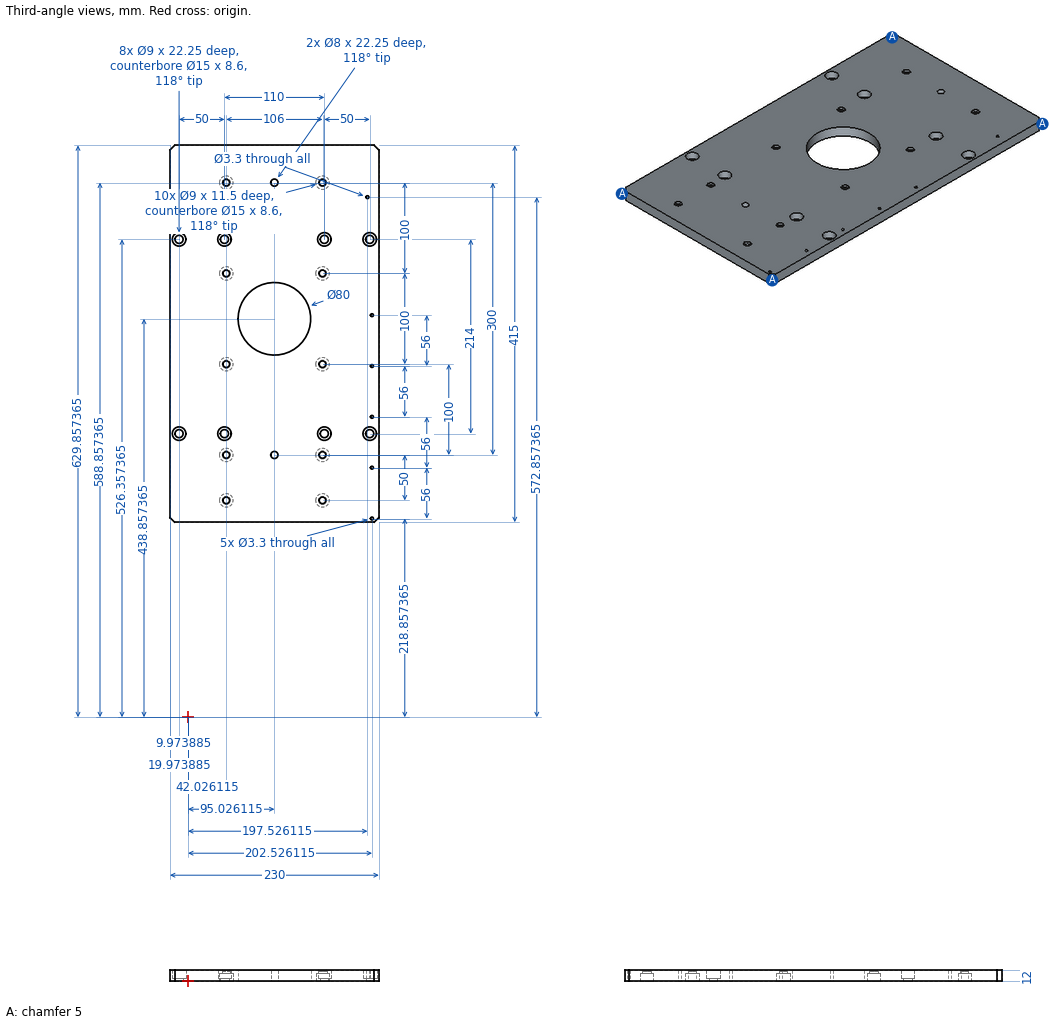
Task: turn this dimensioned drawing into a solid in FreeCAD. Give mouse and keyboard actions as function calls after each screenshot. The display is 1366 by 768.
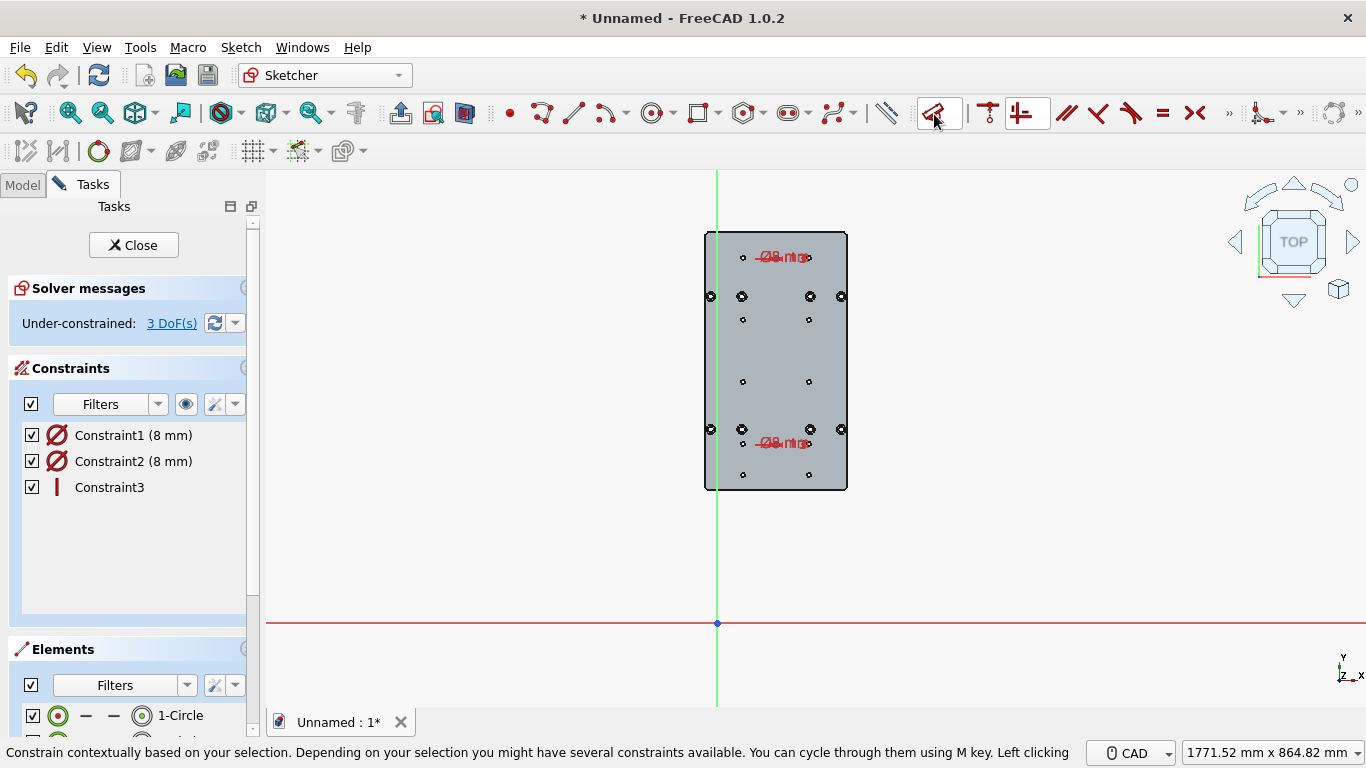
click(776, 259)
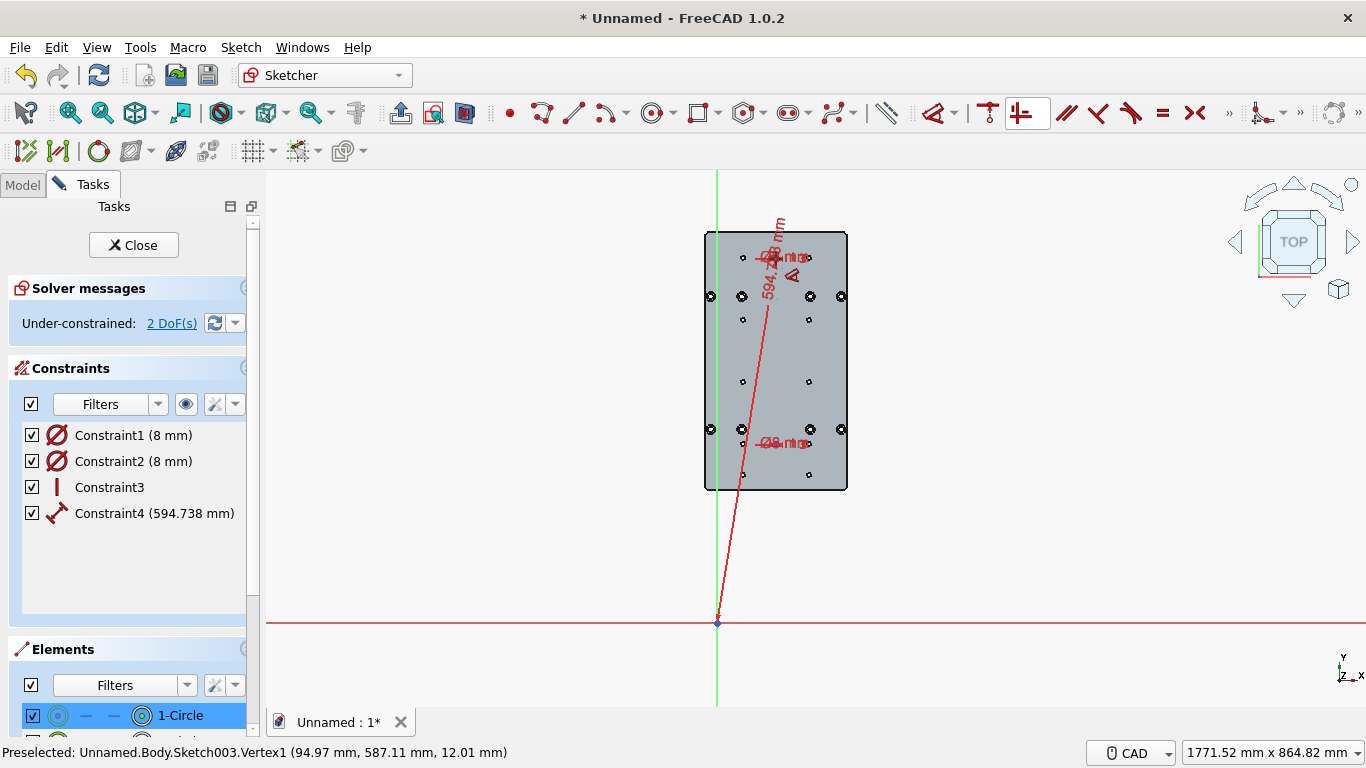
click(776, 445)
click(810, 352)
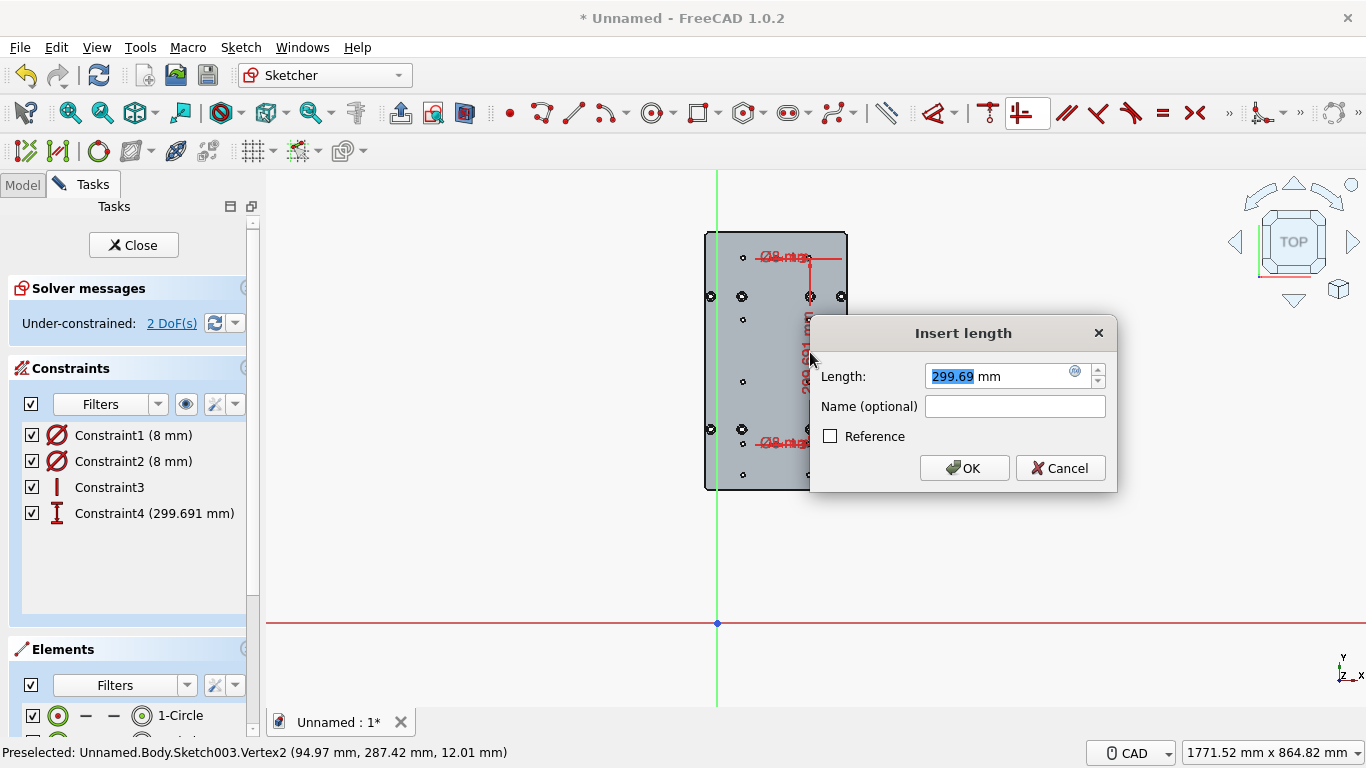
text(300)
key(Return)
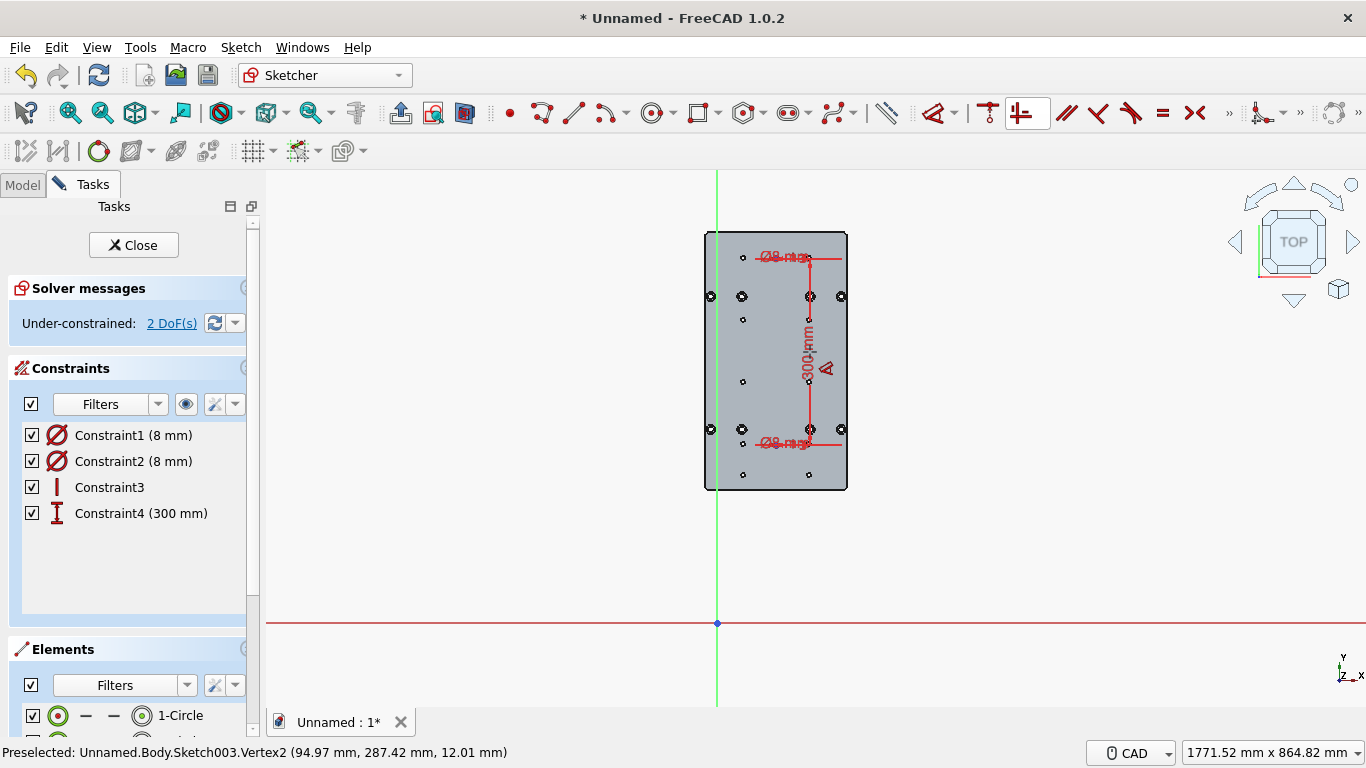
click(776, 259)
click(747, 657)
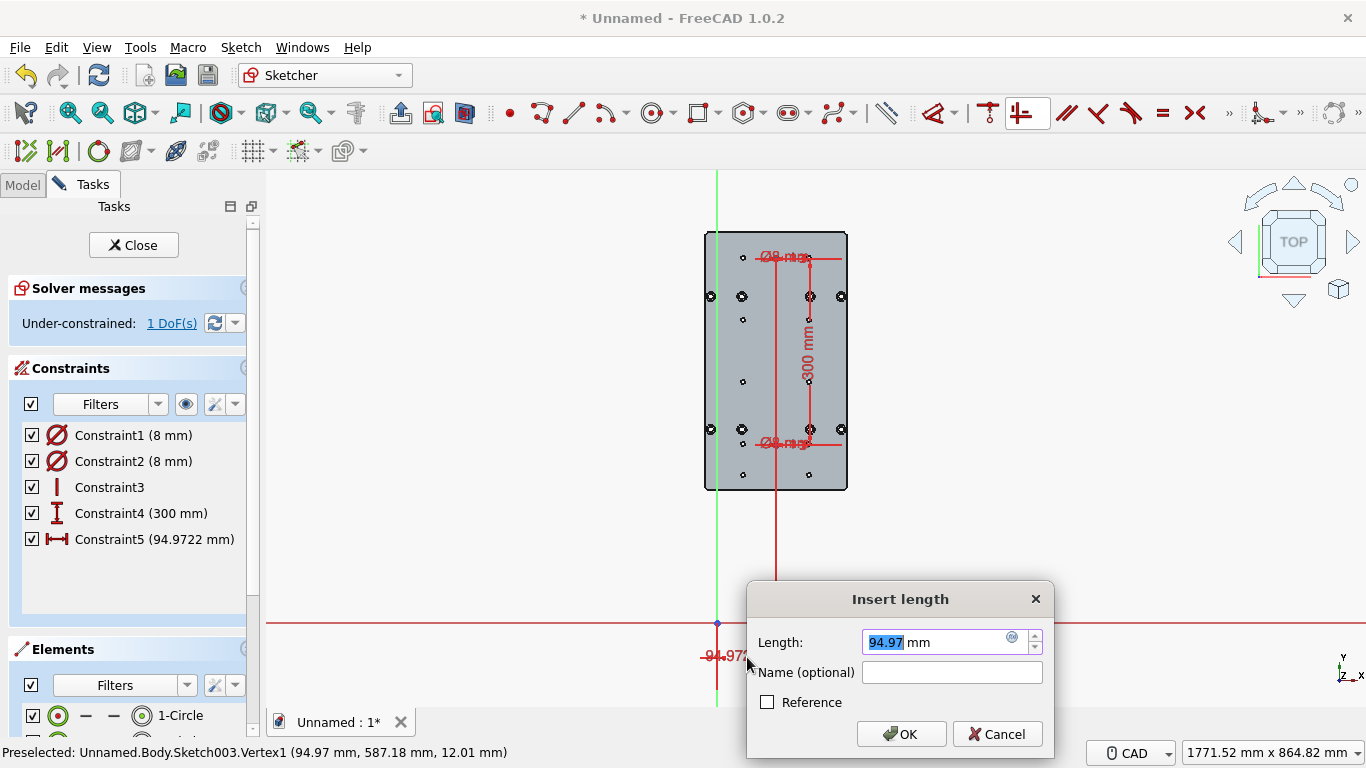
text(95.026115)
key(Return)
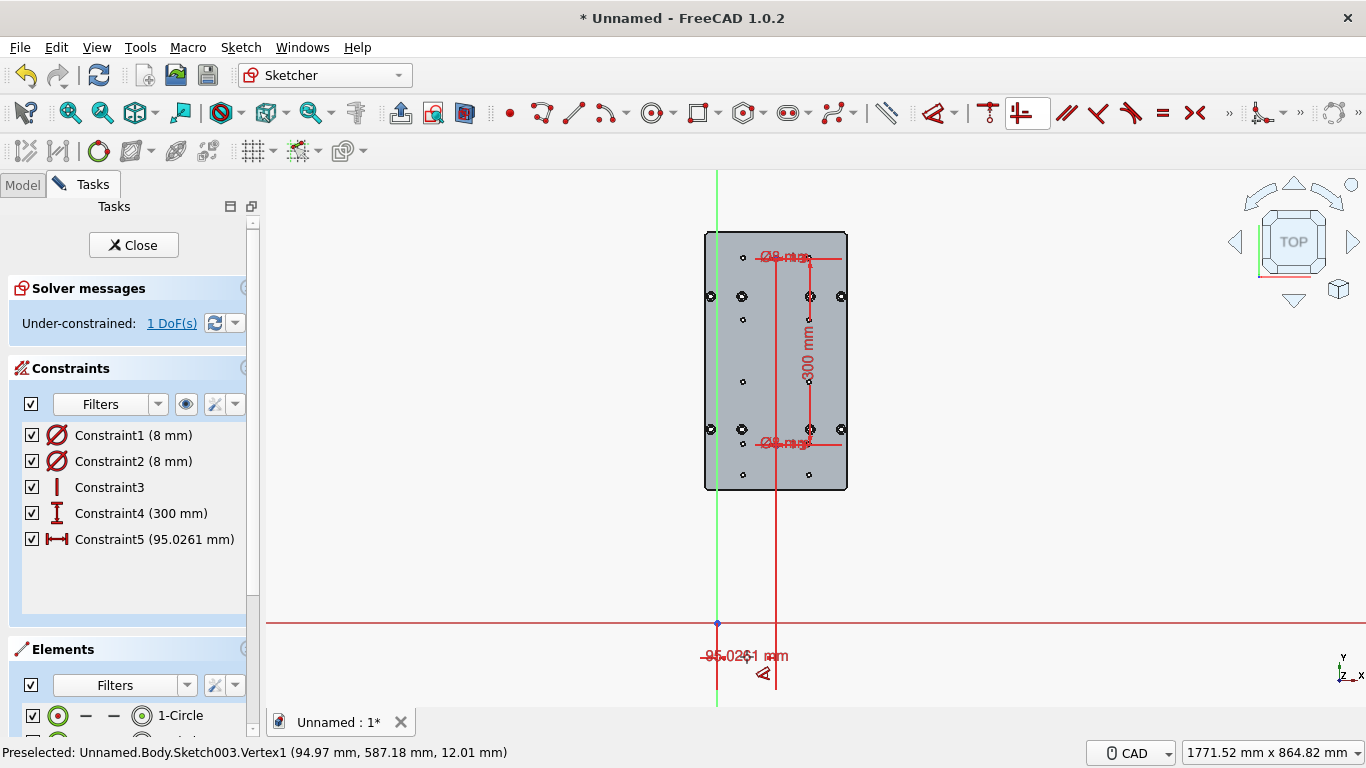
click(776, 259)
click(683, 441)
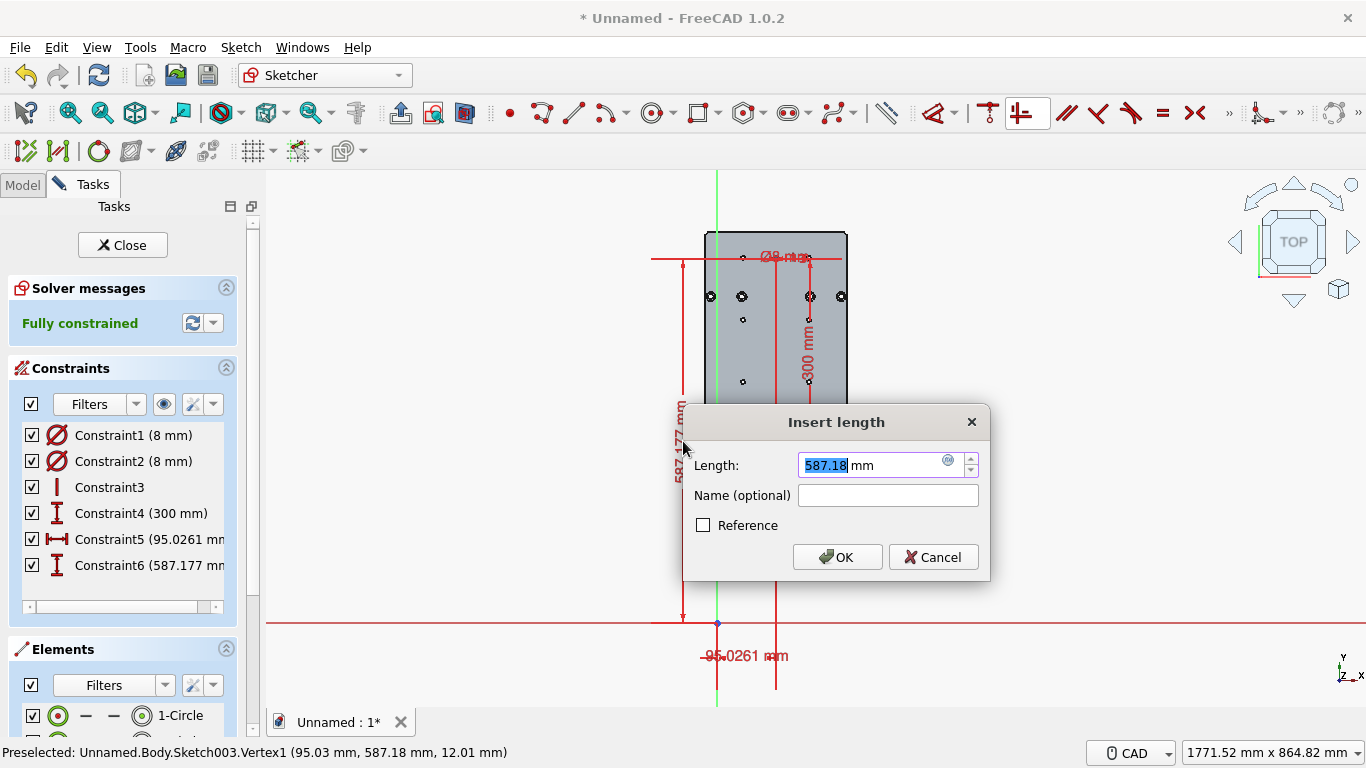
text(588.857365)
key(Return)
key(Escape)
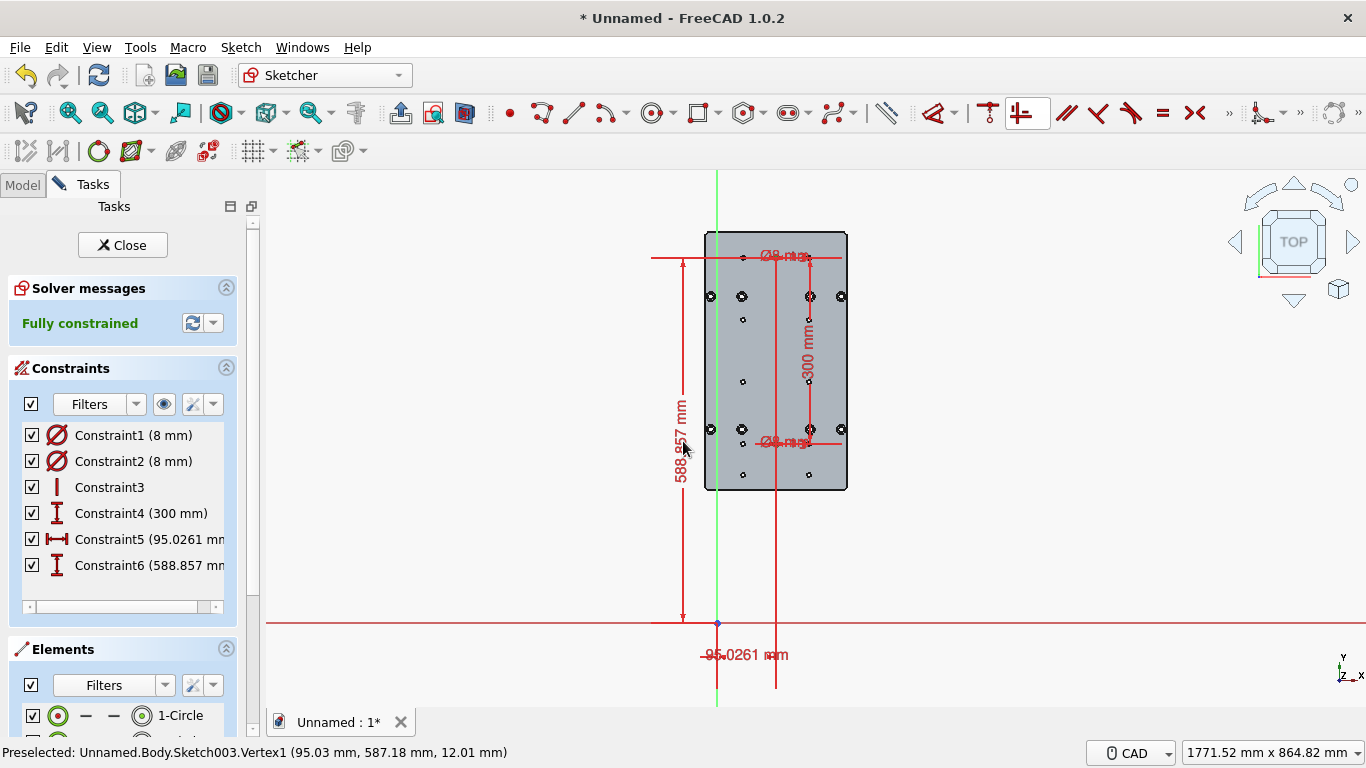
click(123, 245)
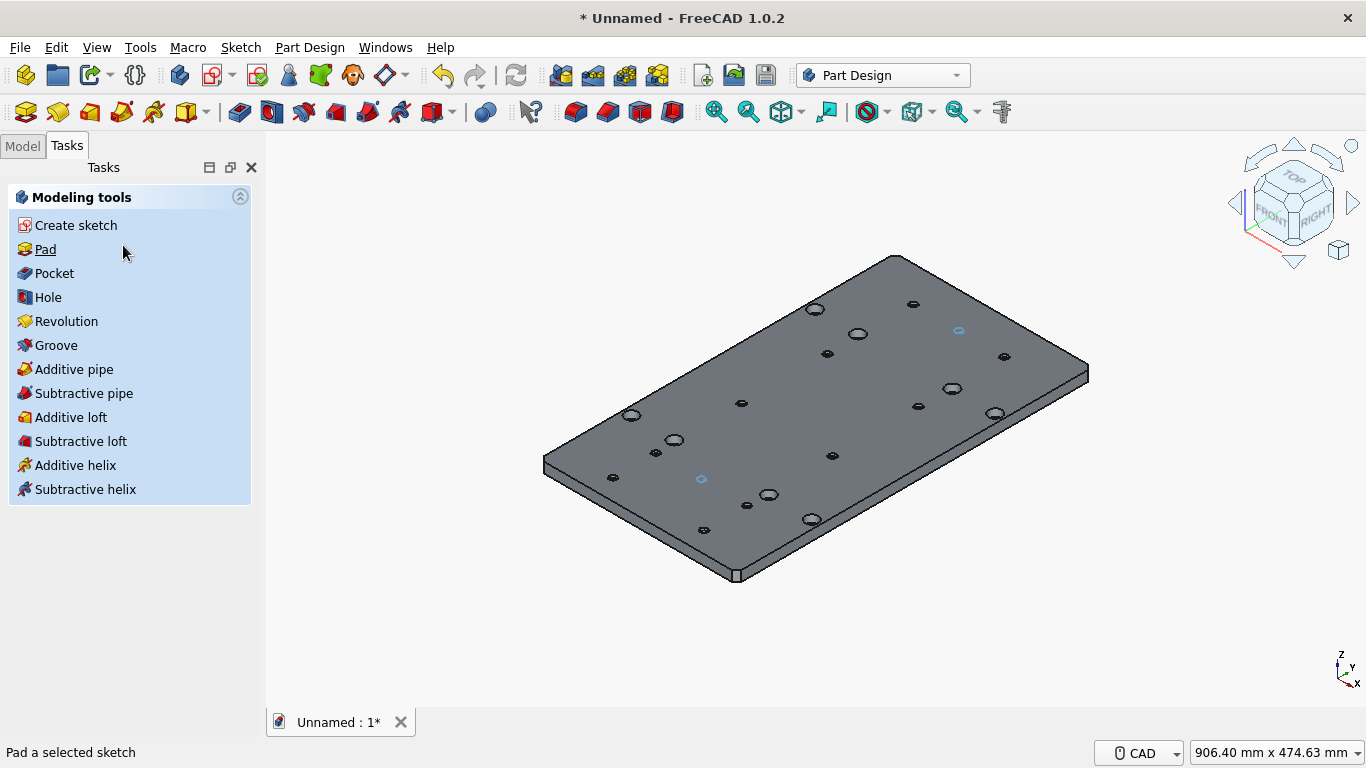
click(272, 112)